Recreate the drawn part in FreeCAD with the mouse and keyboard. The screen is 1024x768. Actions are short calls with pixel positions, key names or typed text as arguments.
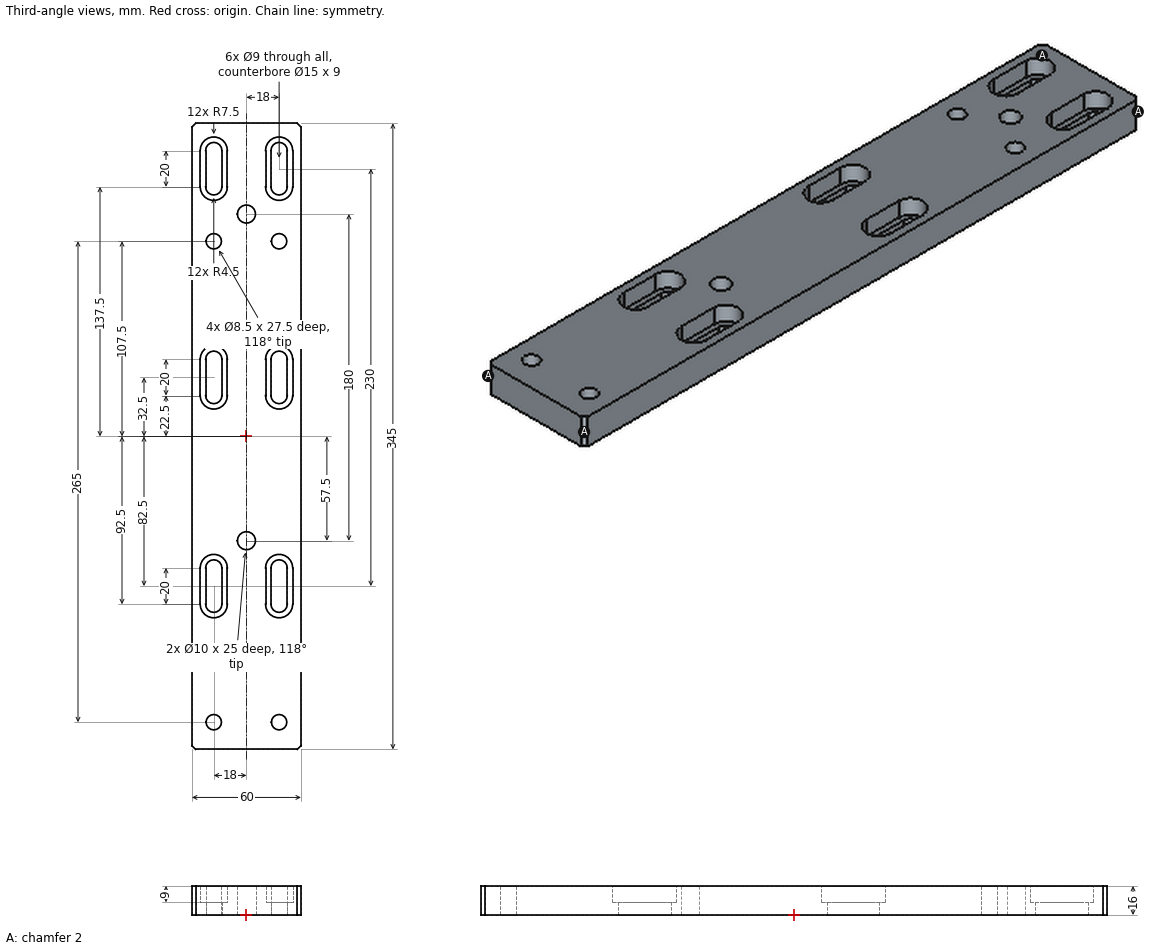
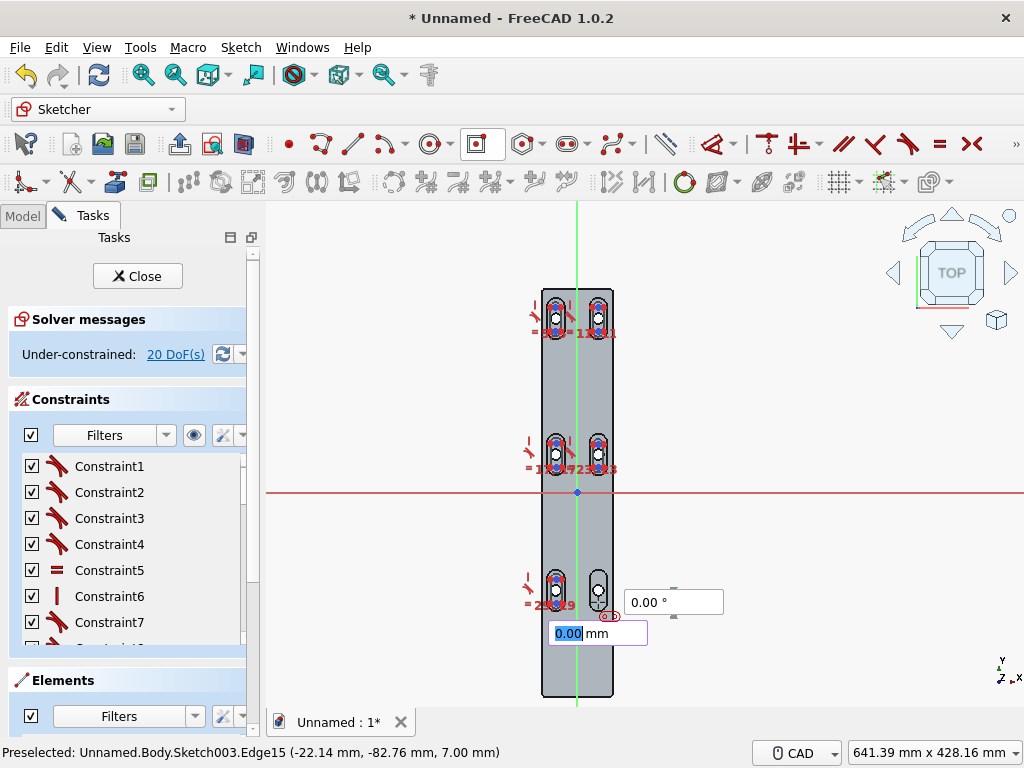
click(598, 579)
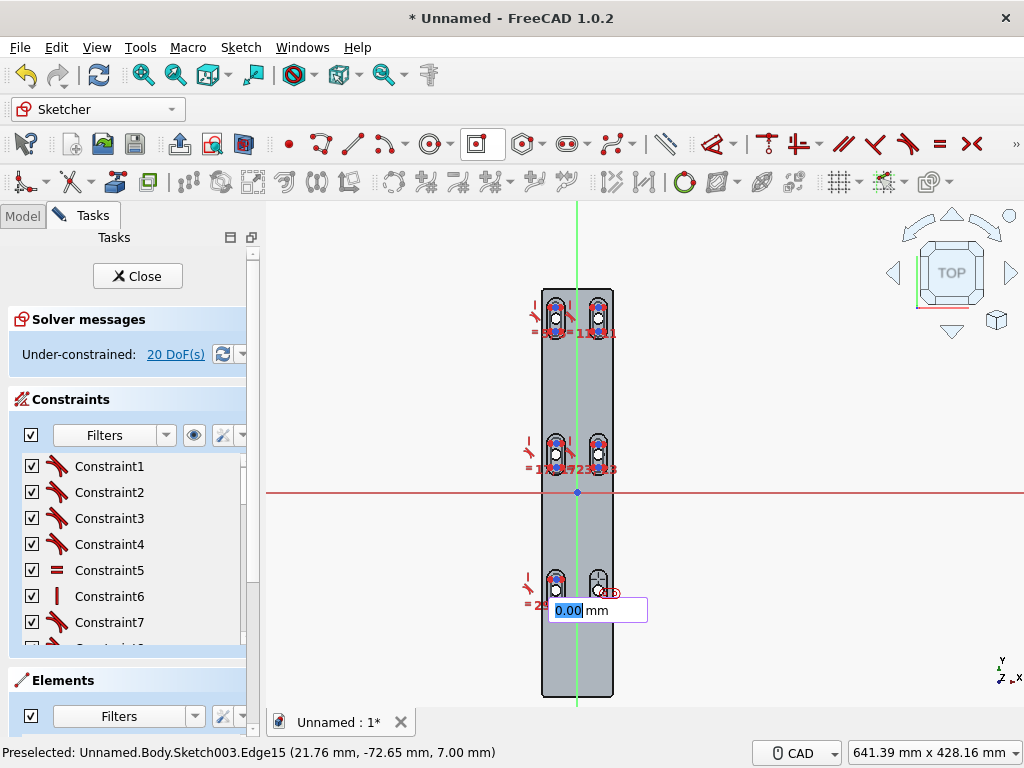
scroll(593, 590, up, 6)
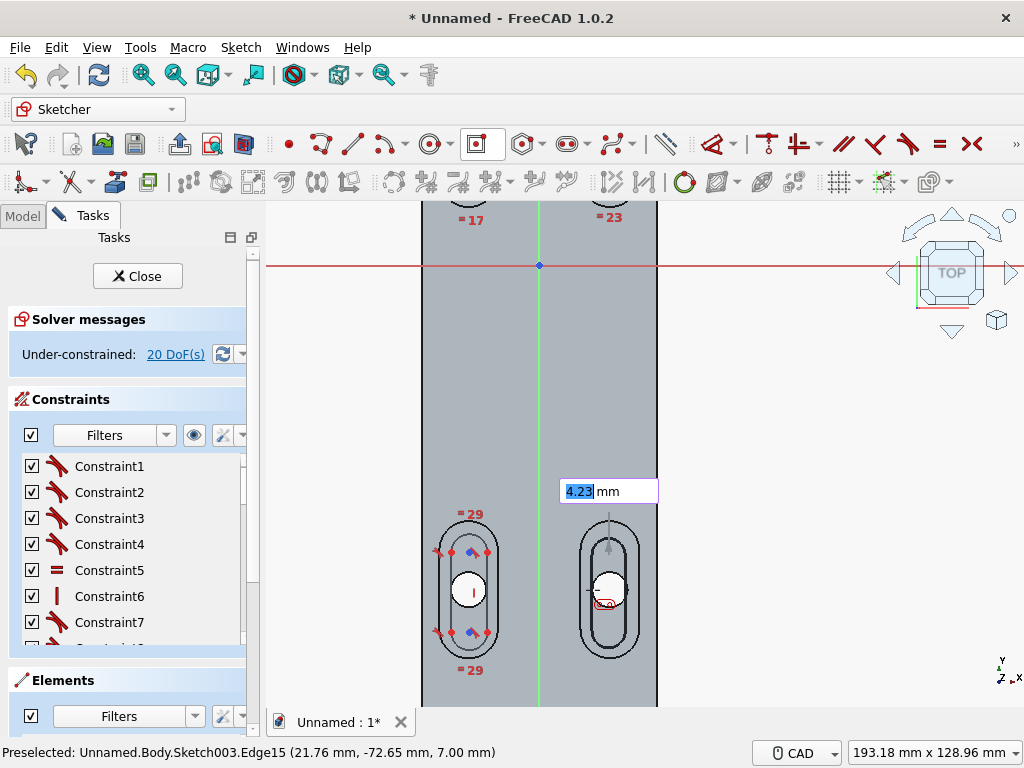
click(592, 590)
key(Escape)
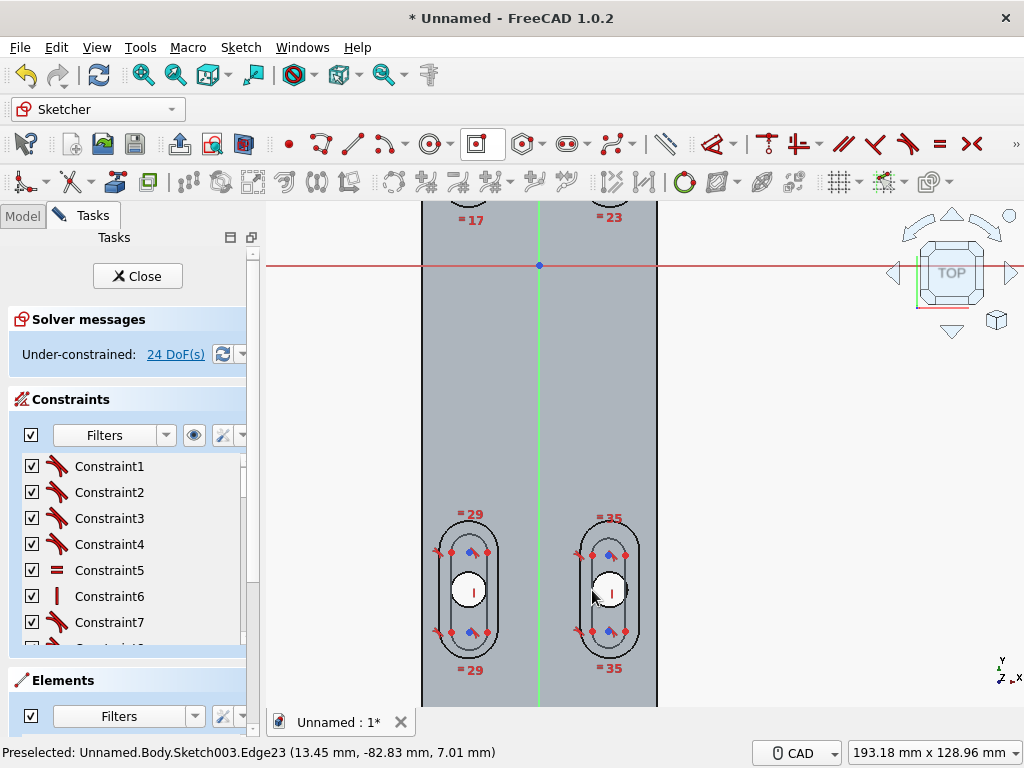
scroll(593, 590, down, 6)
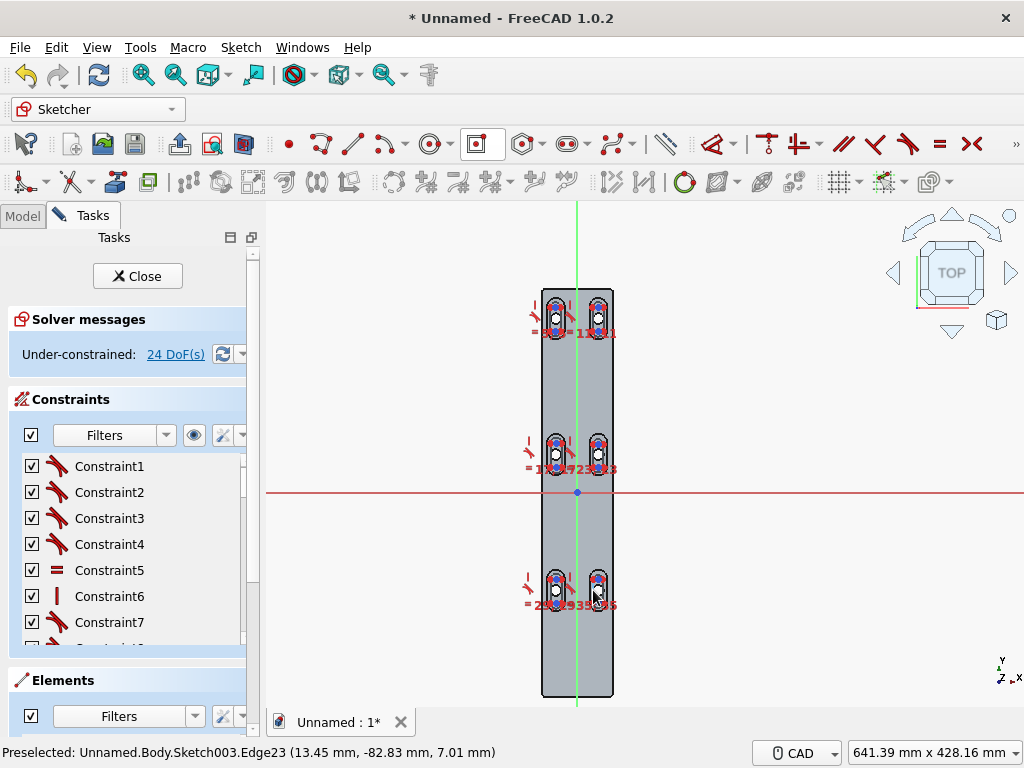
scroll(553, 335, up, 6)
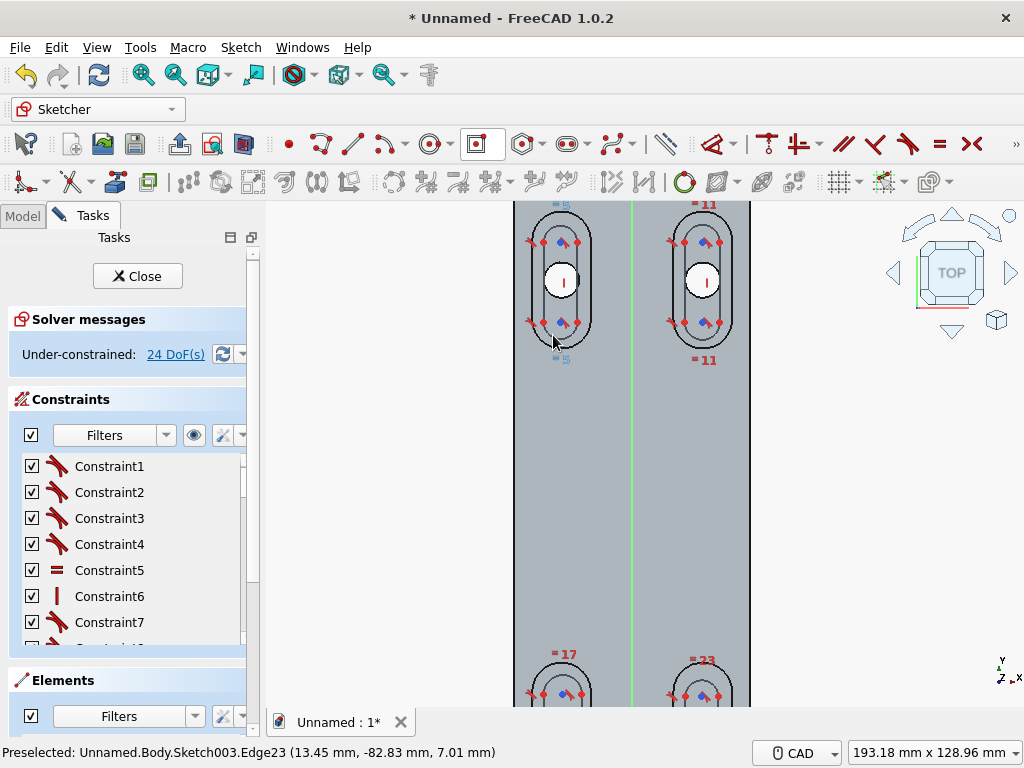
click(551, 336)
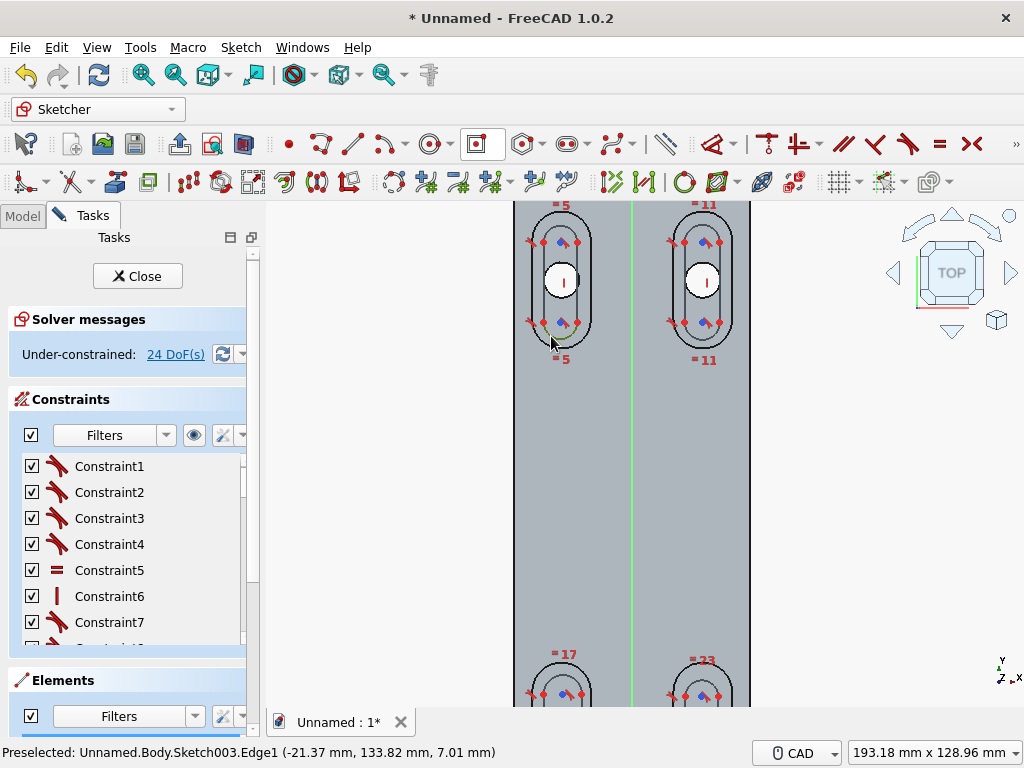
click(692, 336)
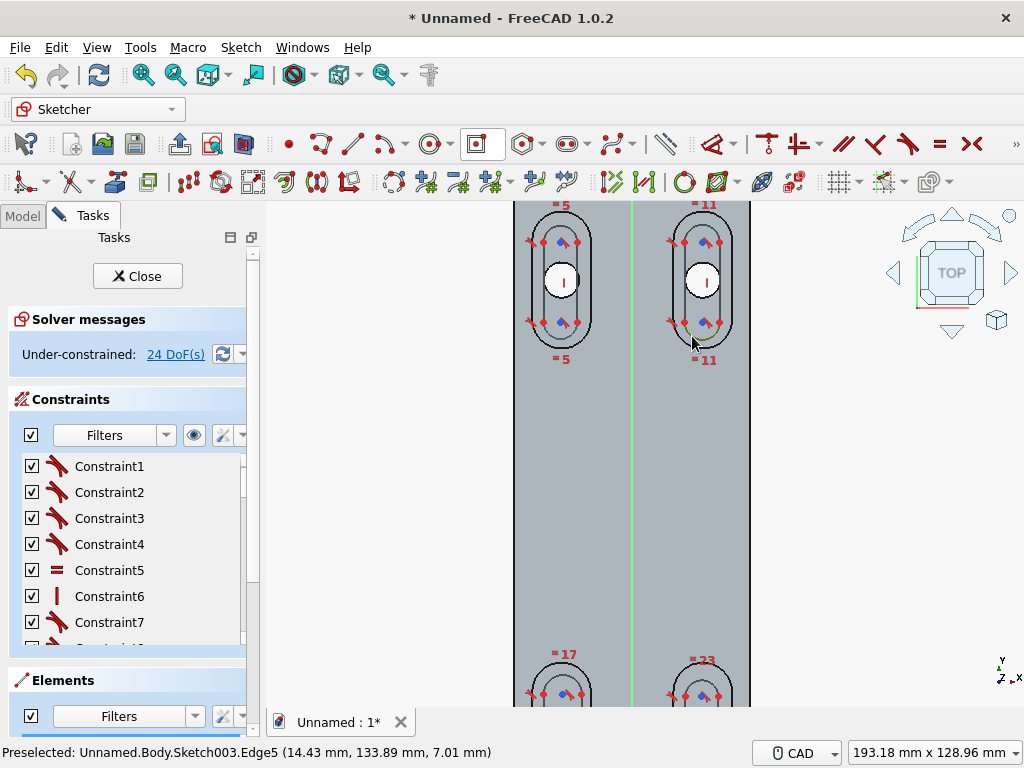
scroll(553, 334, down, 6)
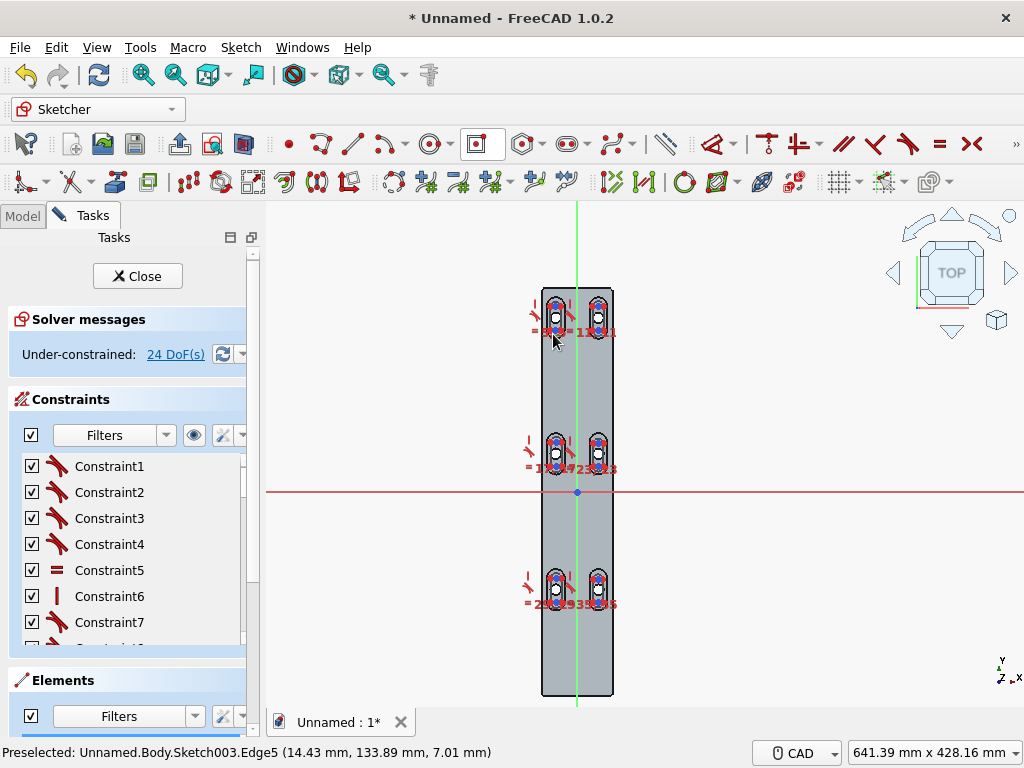
scroll(553, 471, up, 5)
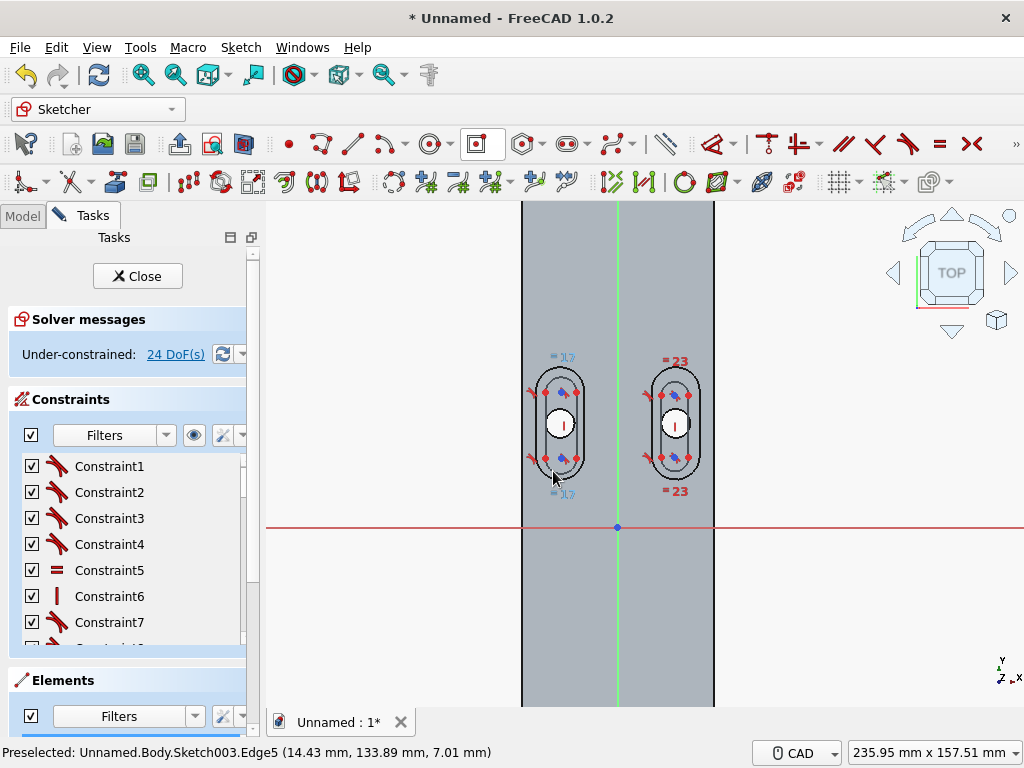
click(552, 471)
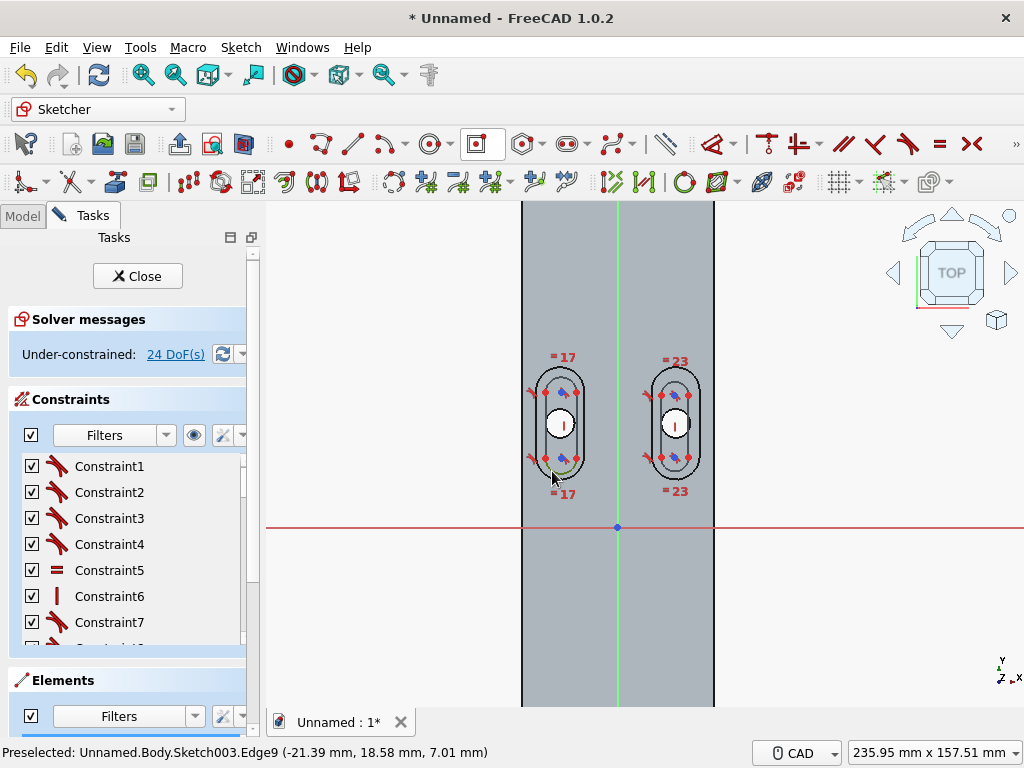
click(667, 469)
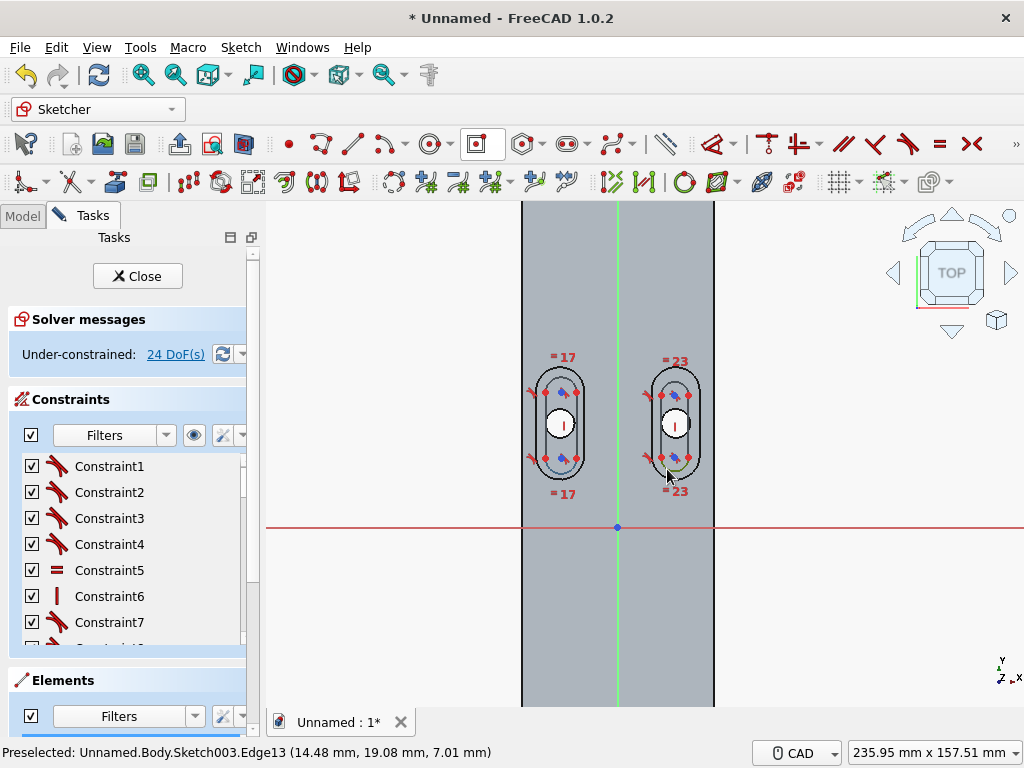
scroll(552, 472, down, 5)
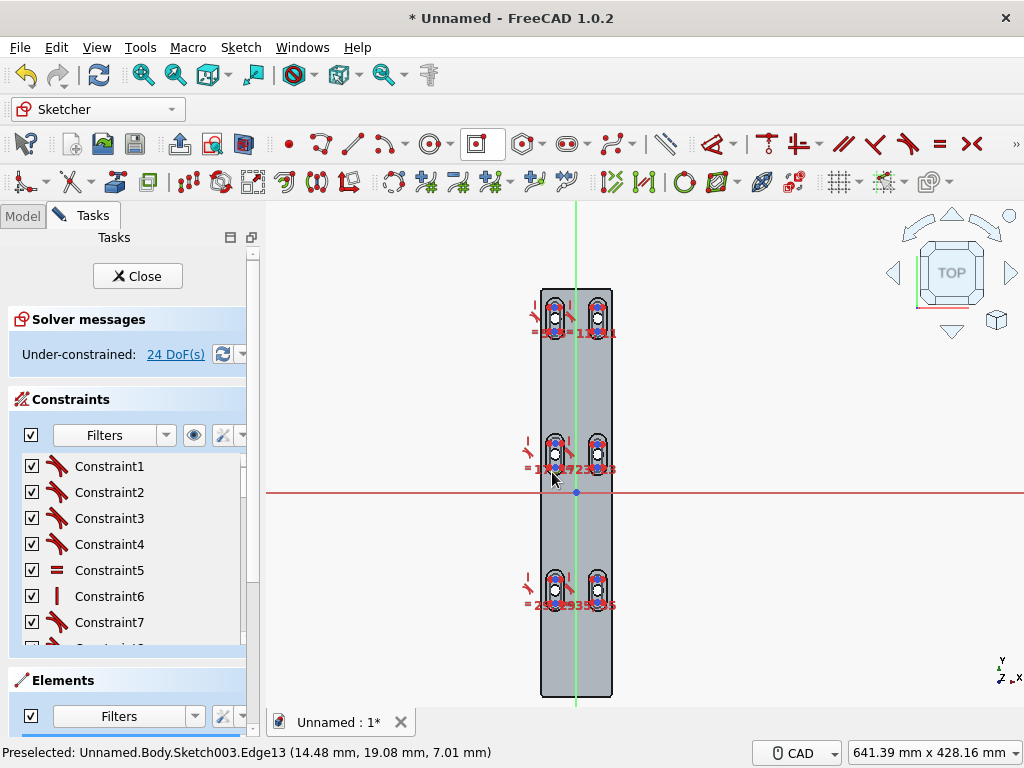
scroll(552, 608, up, 6)